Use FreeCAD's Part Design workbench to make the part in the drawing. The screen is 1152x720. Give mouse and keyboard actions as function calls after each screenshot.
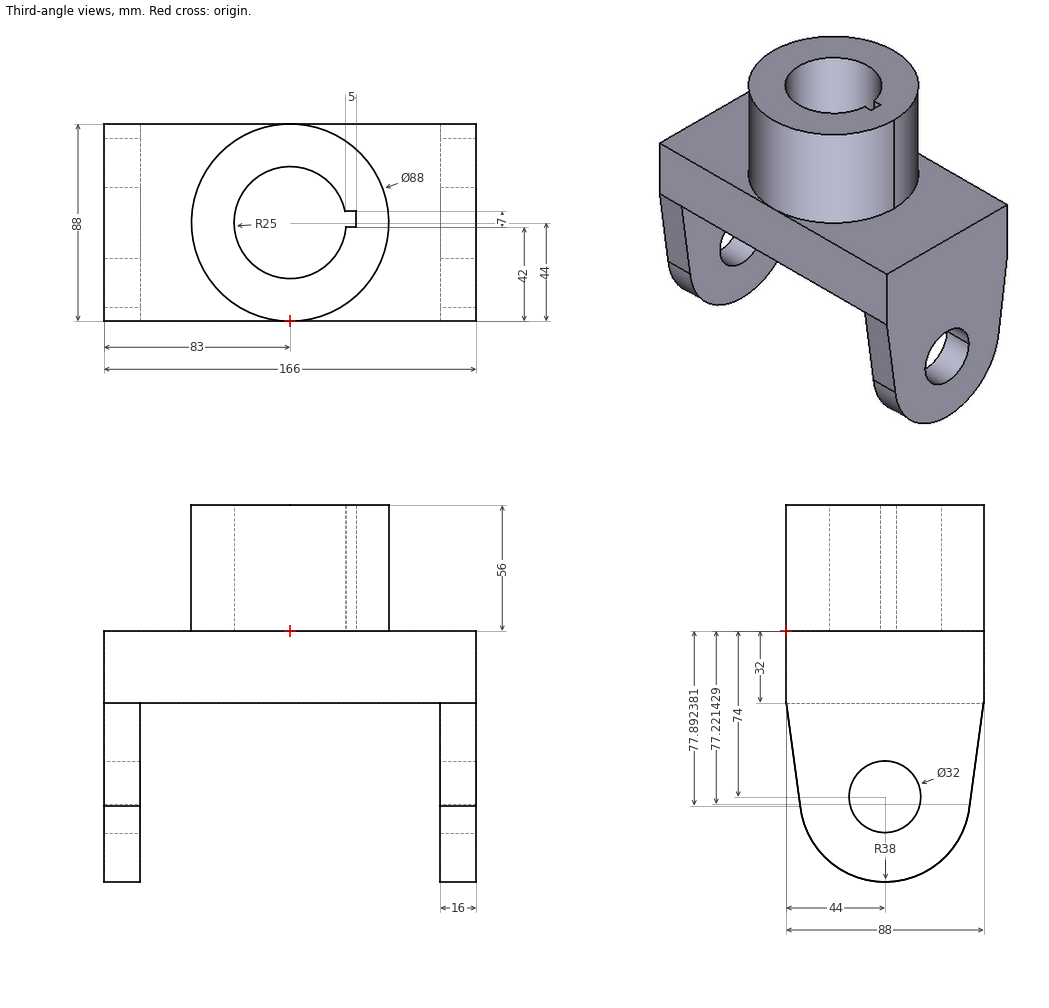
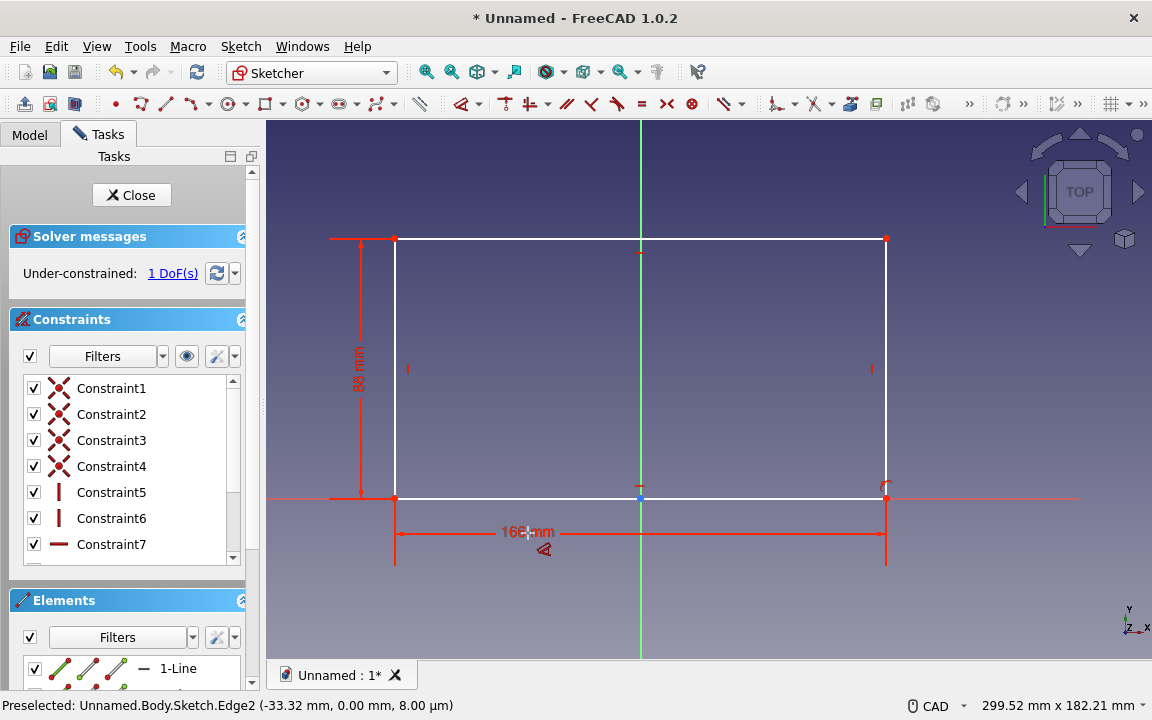
click(395, 239)
click(432, 533)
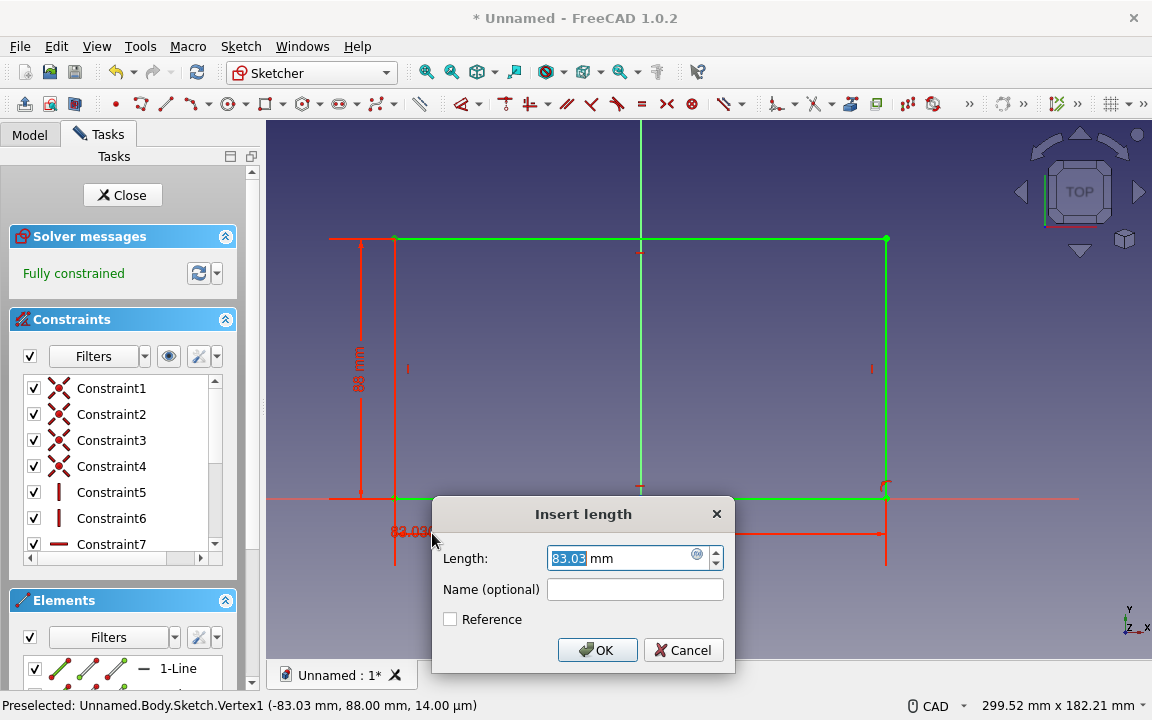
text(83)
key(Return)
key(Escape)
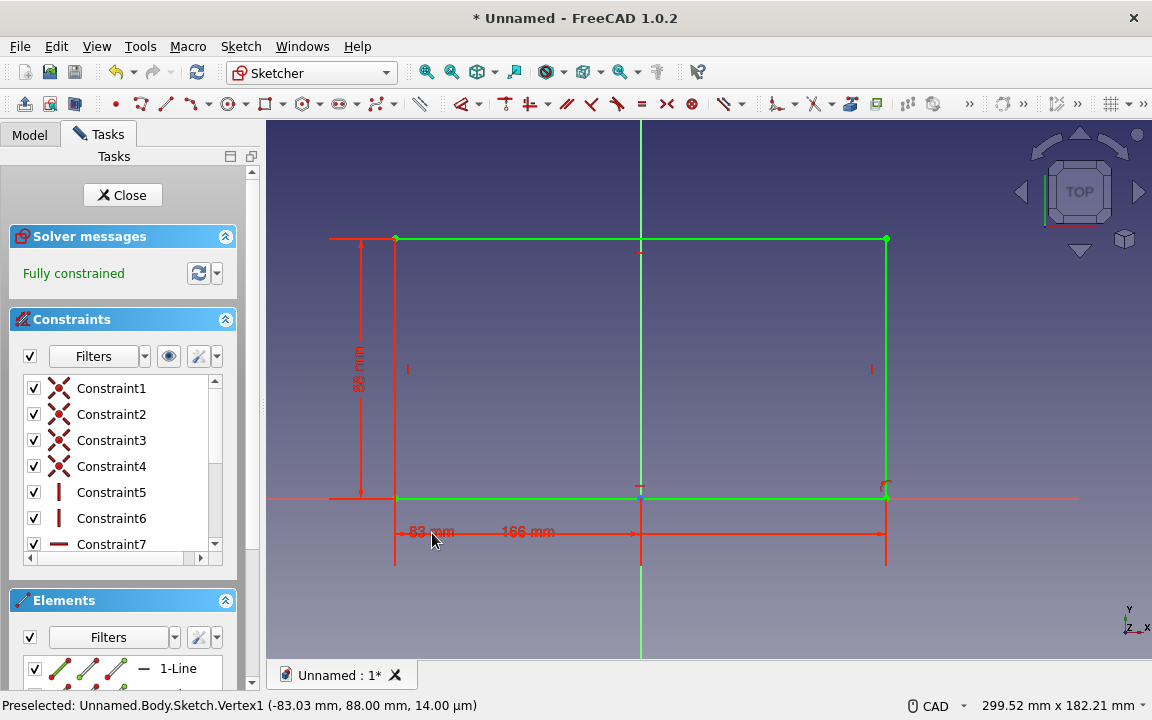
click(123, 195)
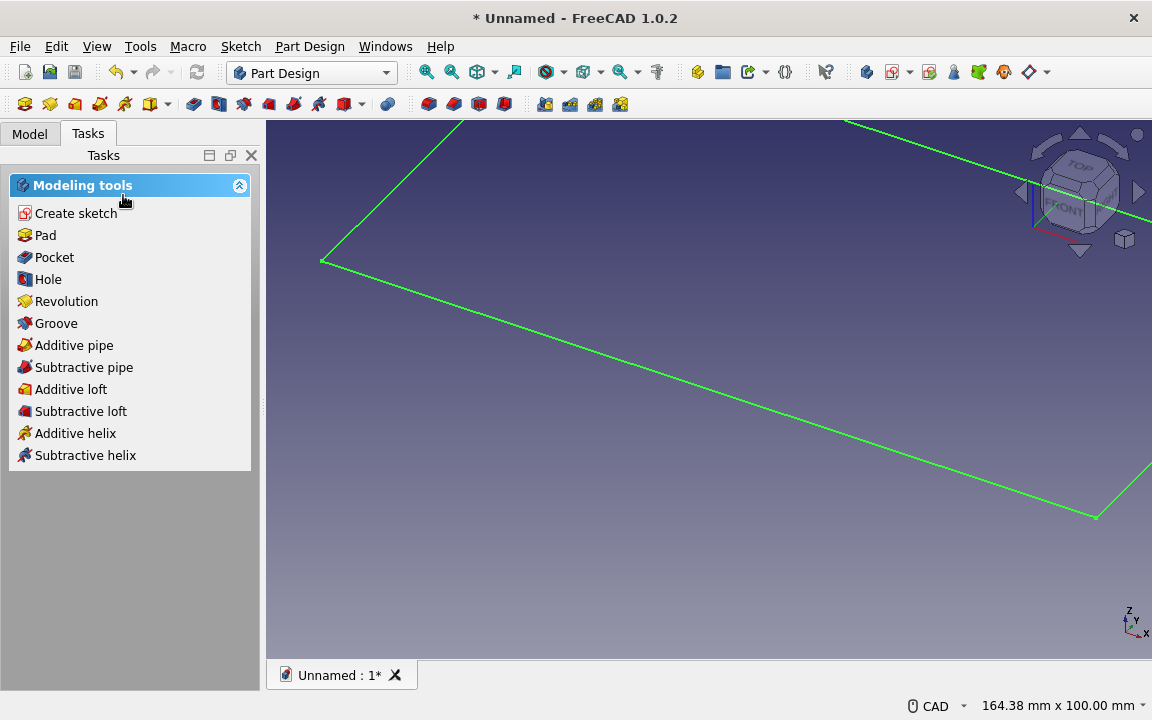
click(25, 104)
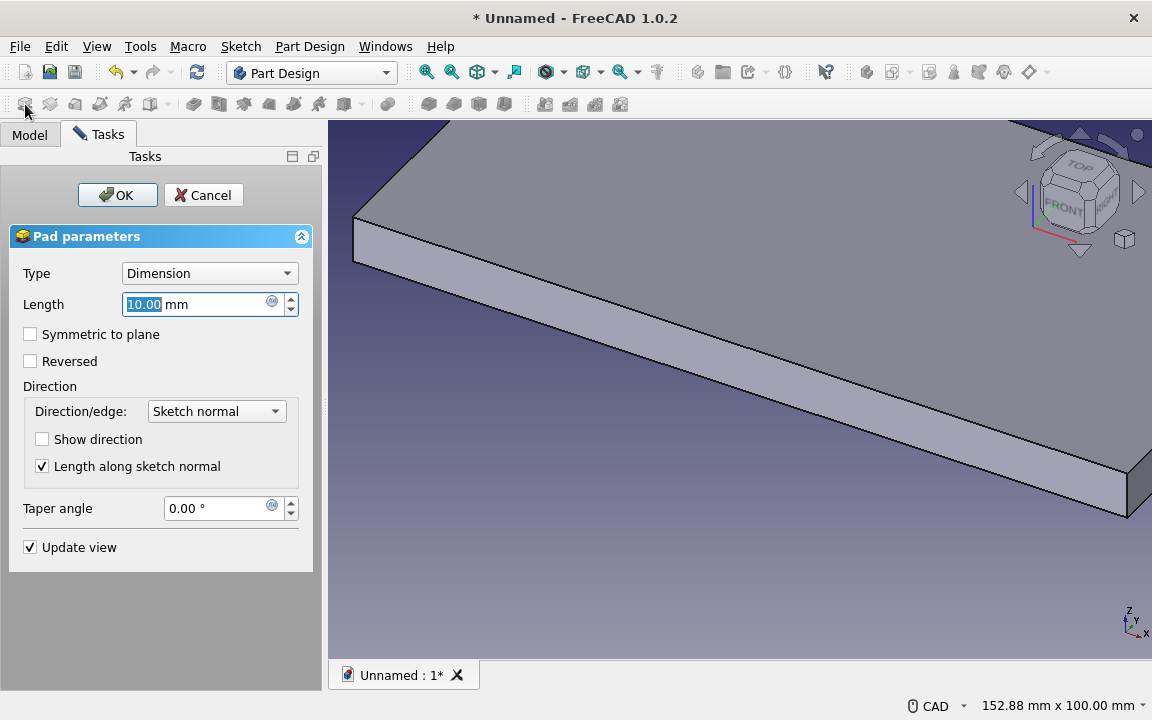
text(32)
key(Tab)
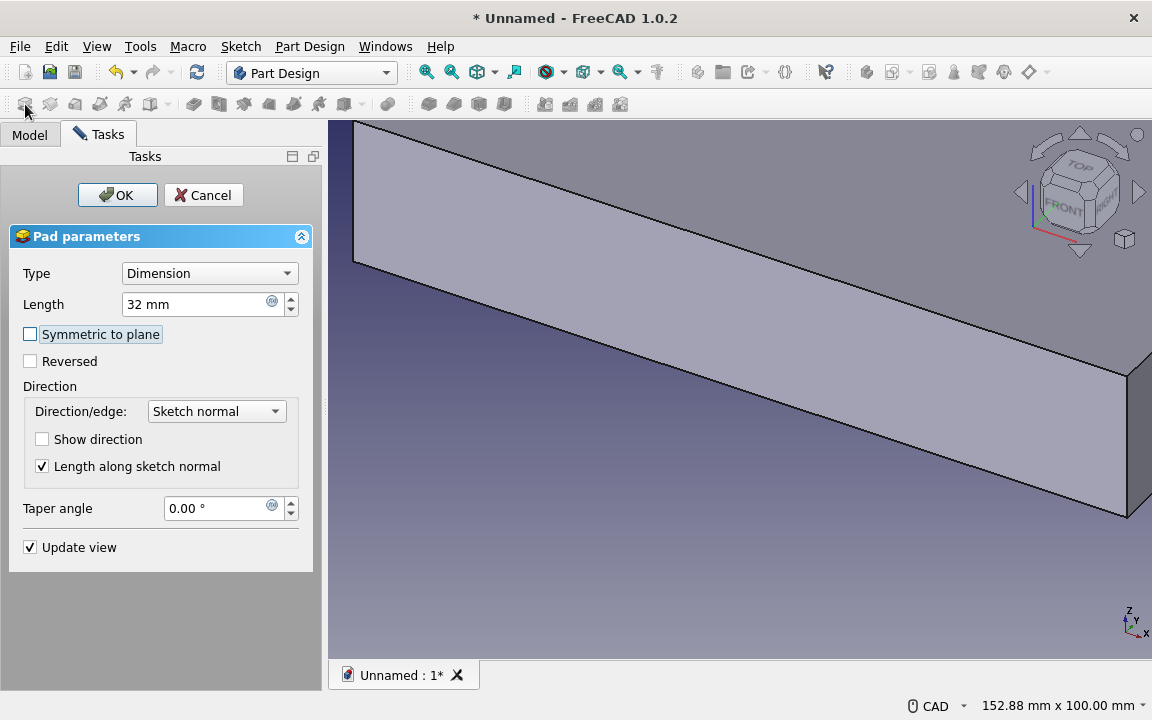
click(31, 361)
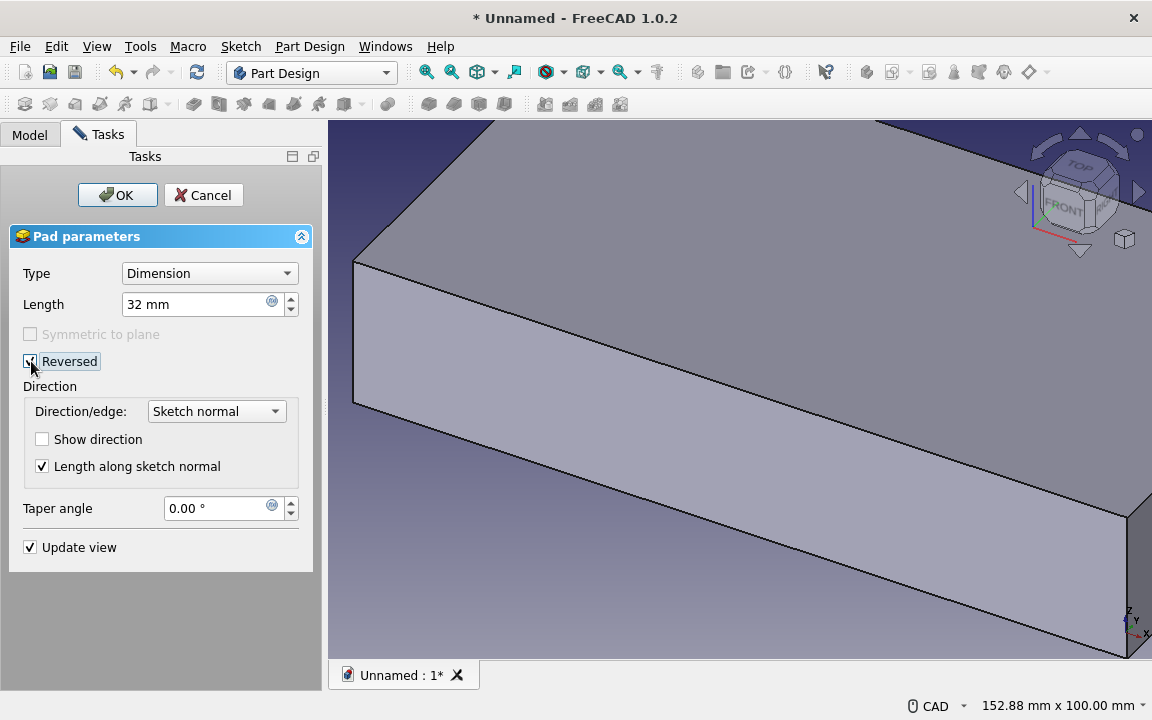
click(118, 195)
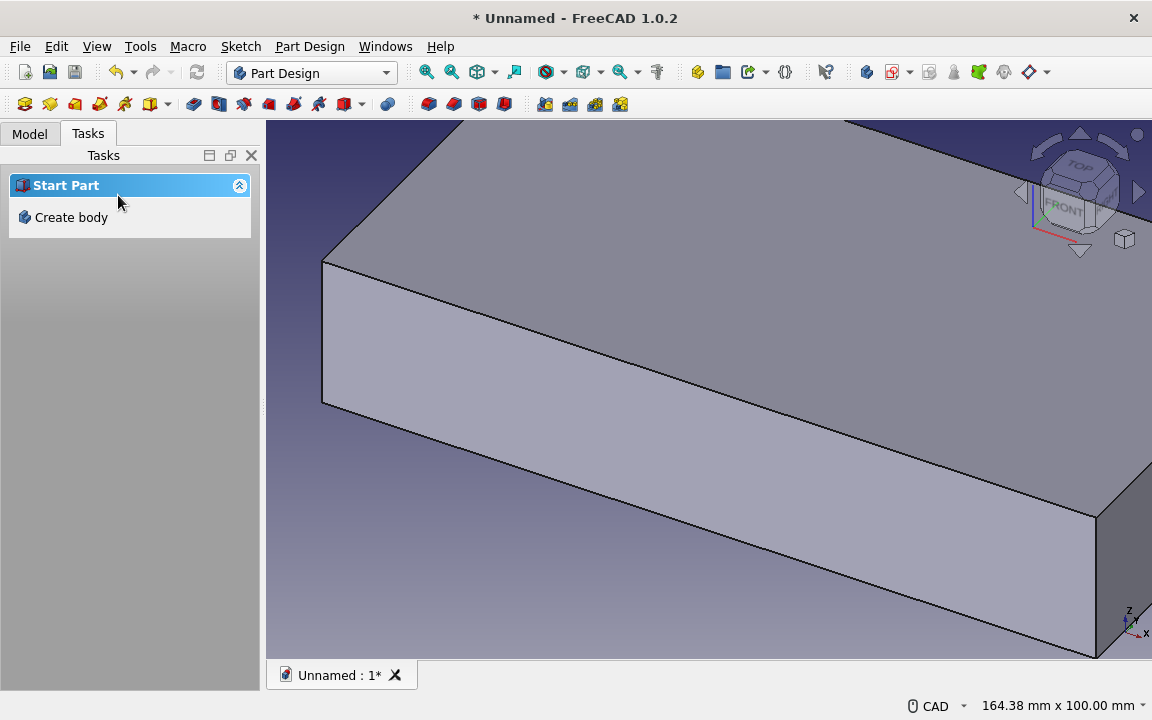
click(427, 72)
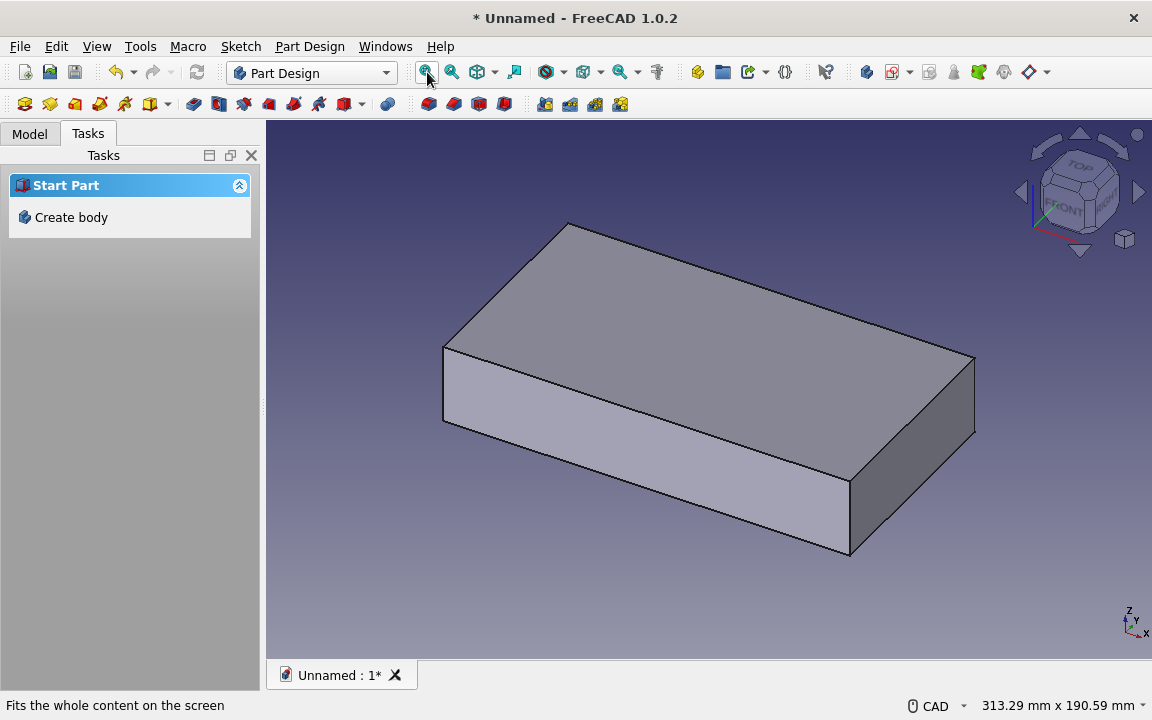
click(948, 420)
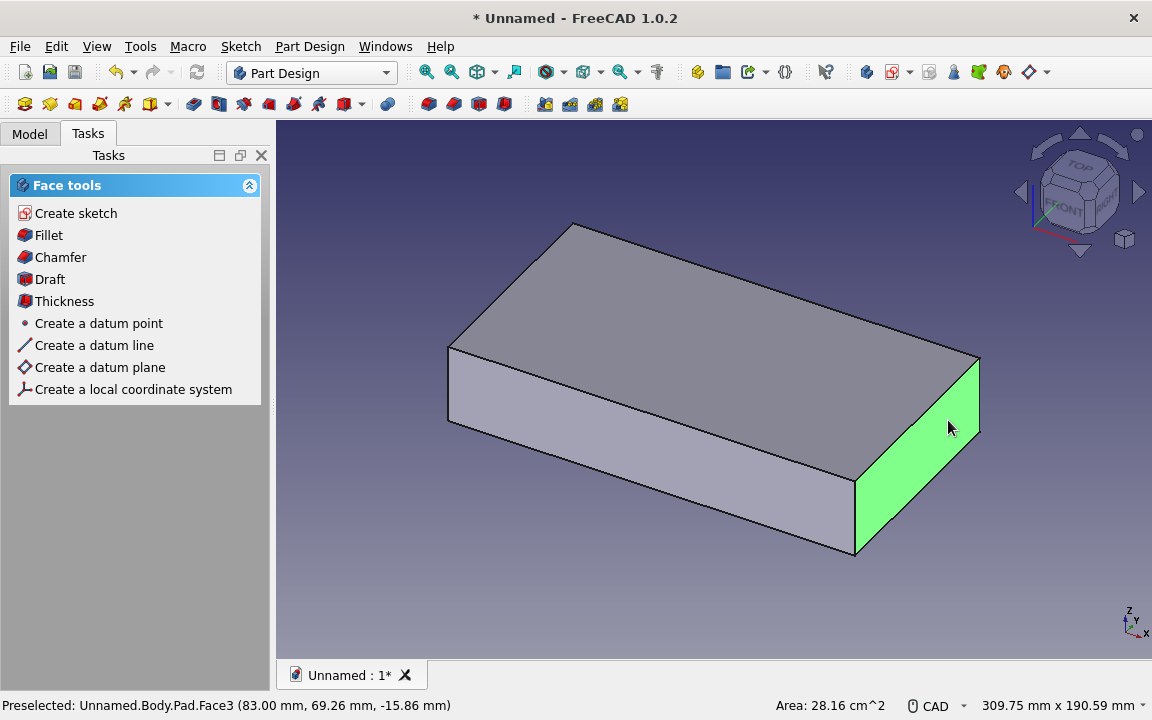
click(892, 72)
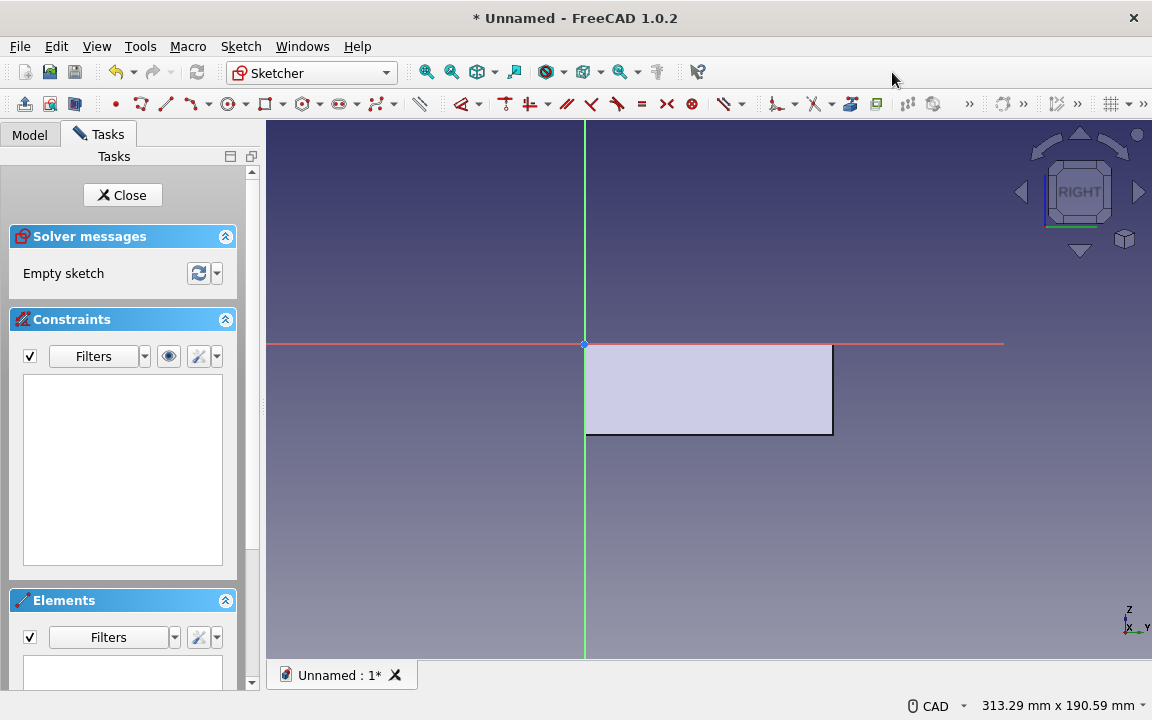
scroll(331, 148, down, 1)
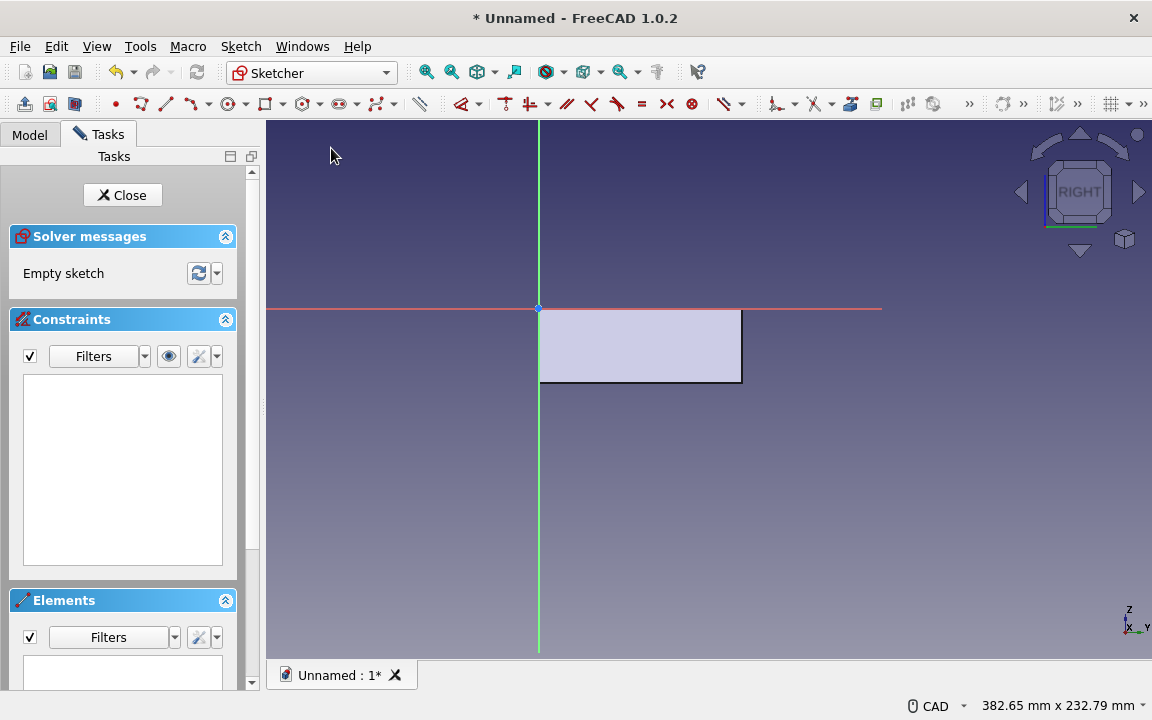
click(141, 104)